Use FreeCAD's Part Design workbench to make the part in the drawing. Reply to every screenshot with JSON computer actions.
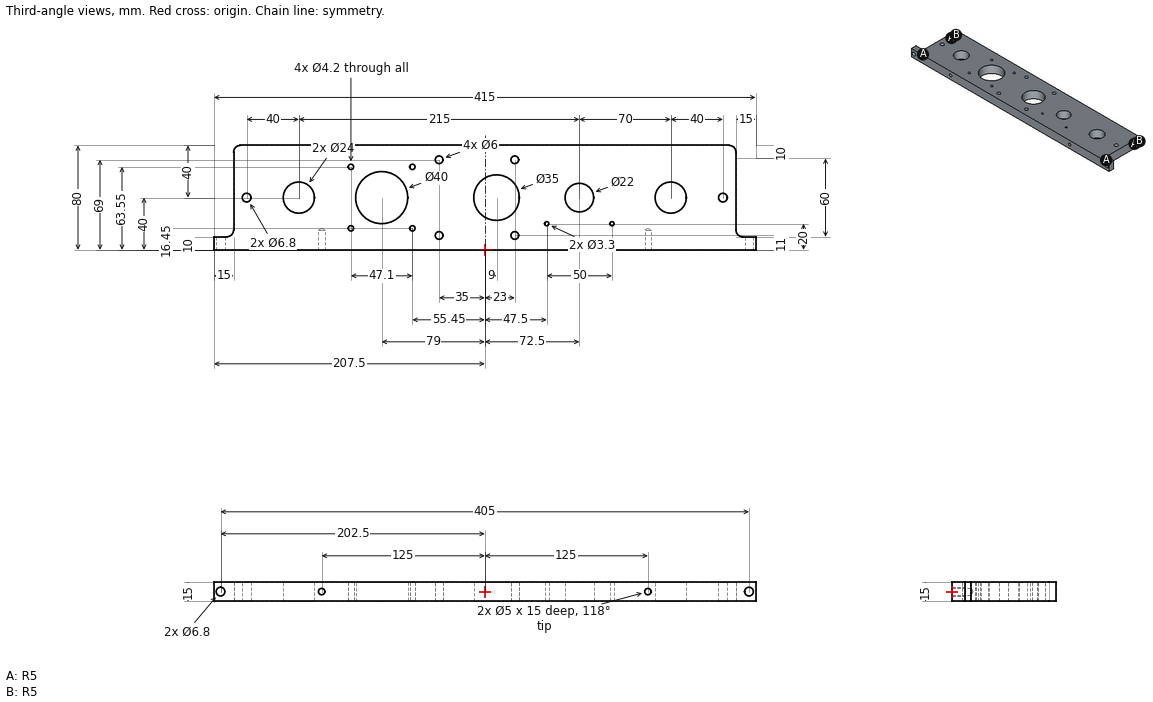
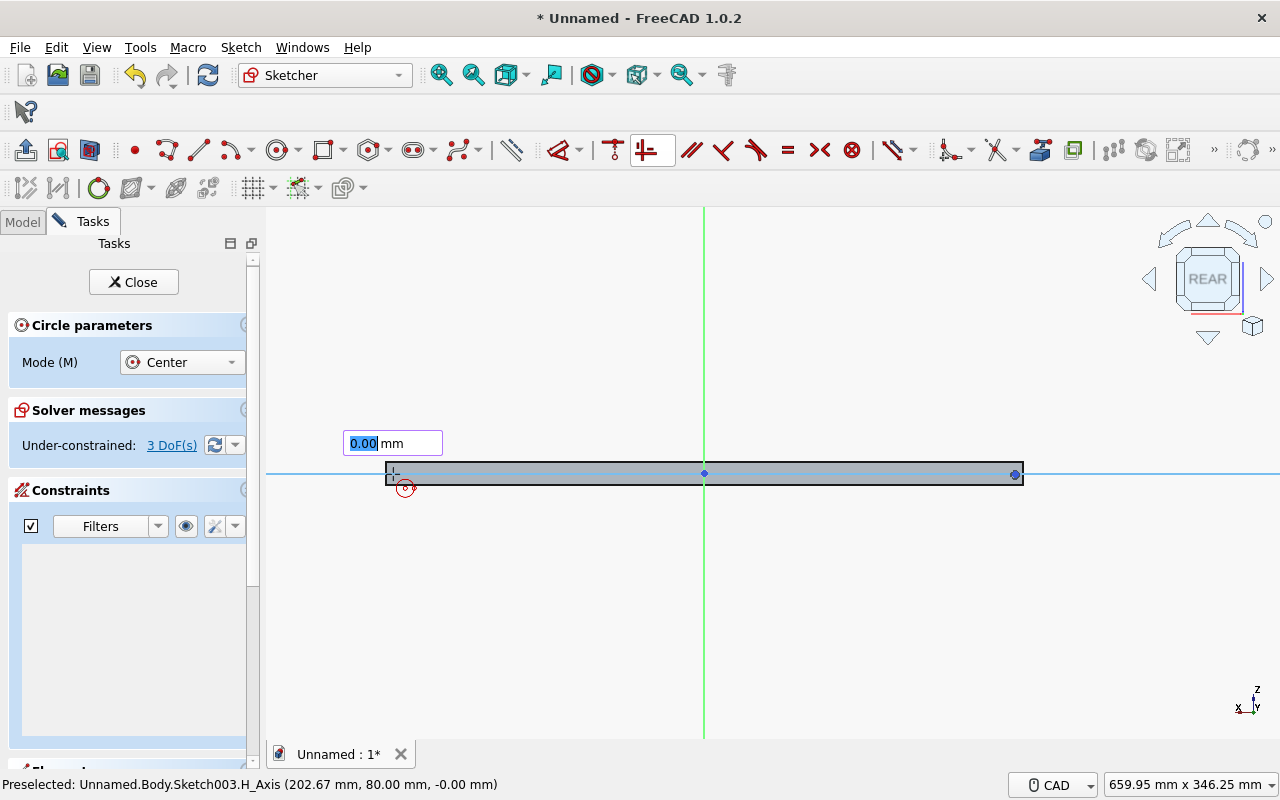
{"action": "scroll", "coordinate": [391, 479], "scroll_direction": "up", "scroll_amount": 6}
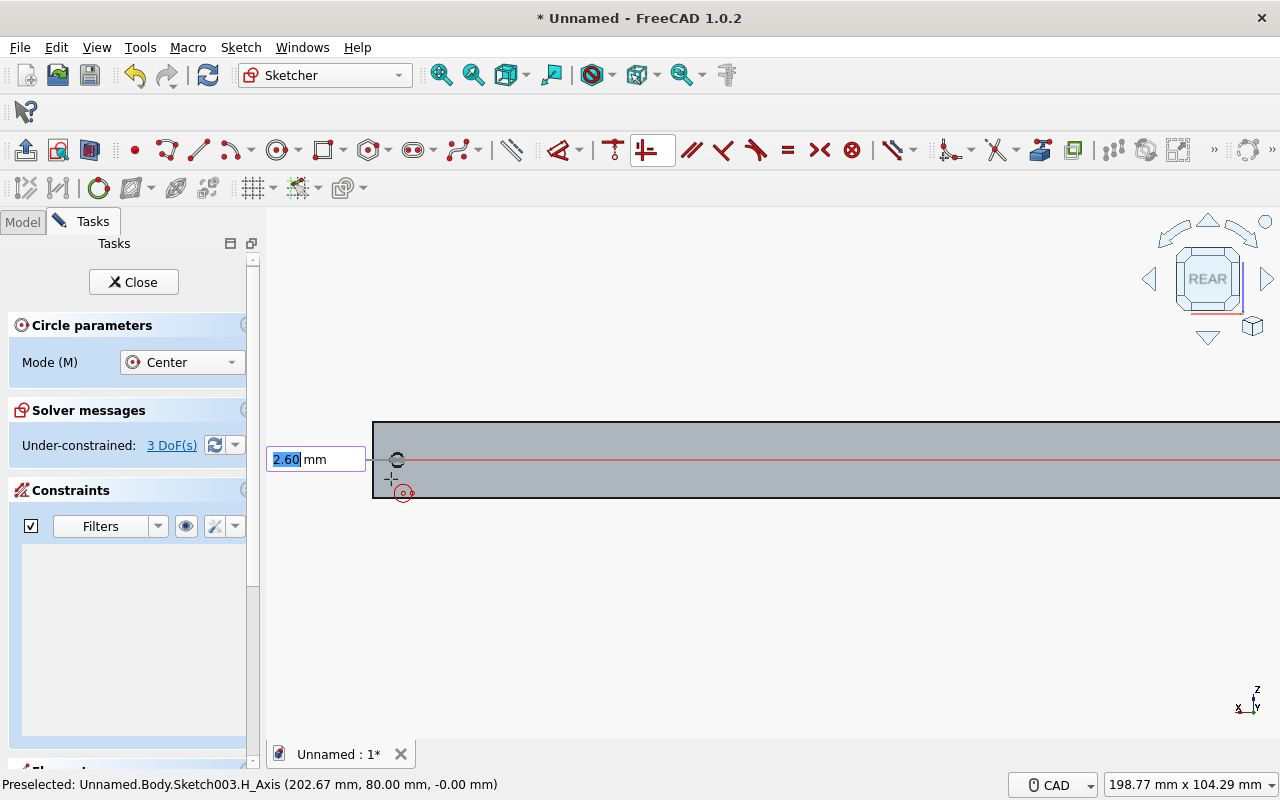
{"action": "left_click", "coordinate": [392, 476]}
{"action": "key", "text": "Escape"}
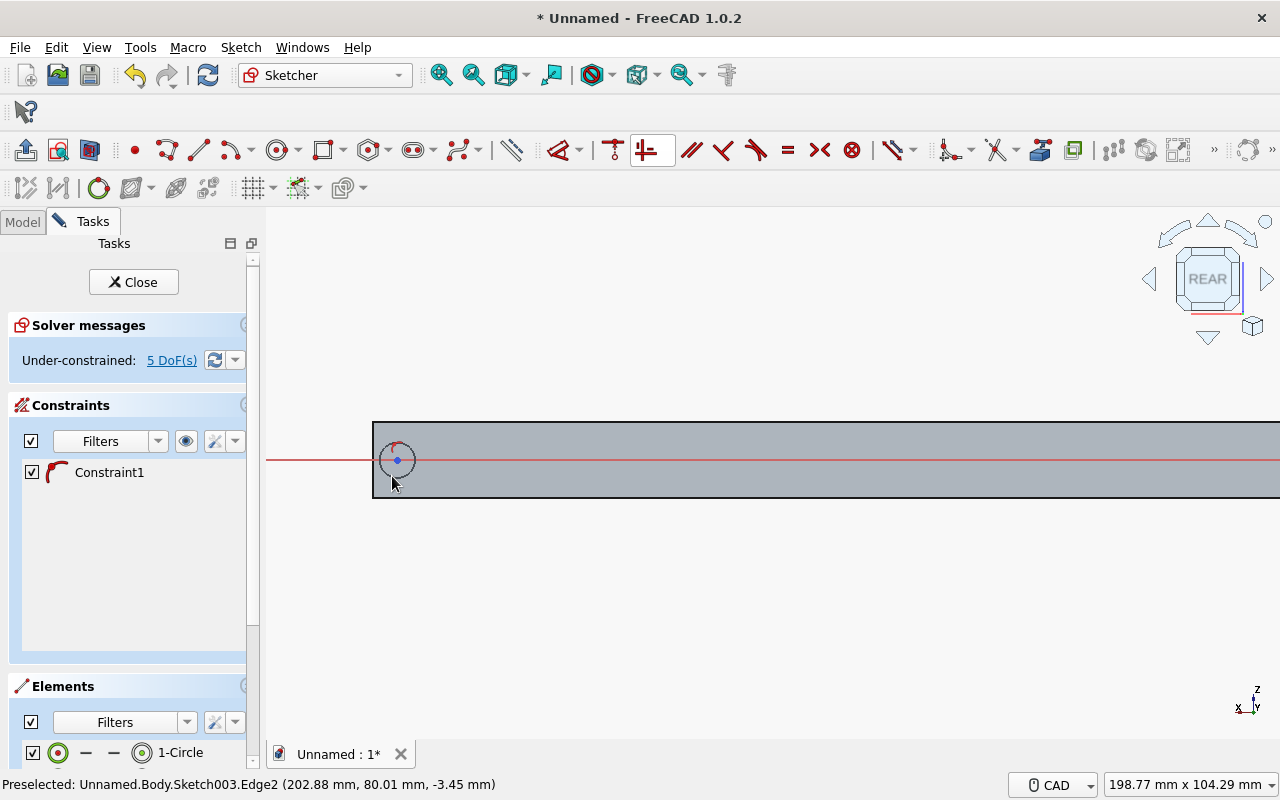
{"action": "scroll", "coordinate": [391, 479], "scroll_direction": "down", "scroll_amount": 6}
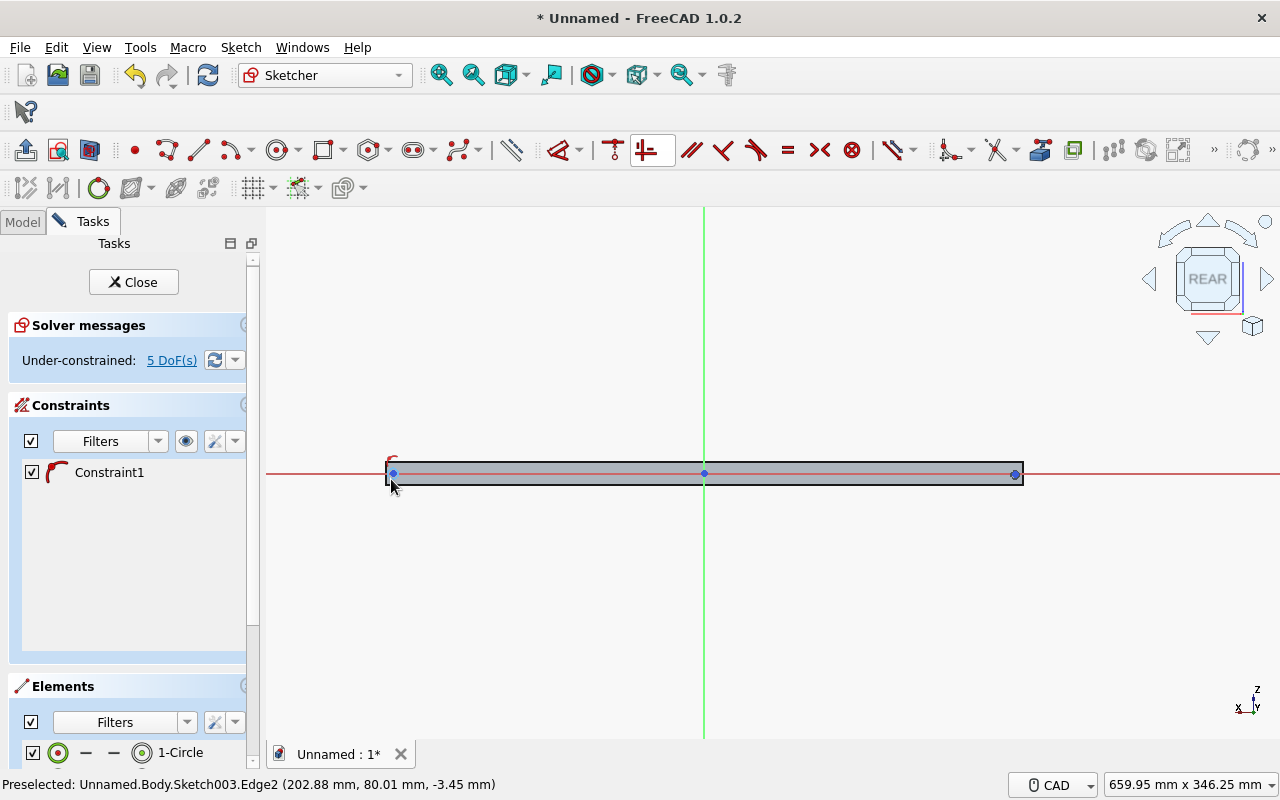
{"action": "scroll", "coordinate": [1012, 478], "scroll_direction": "up", "scroll_amount": 7}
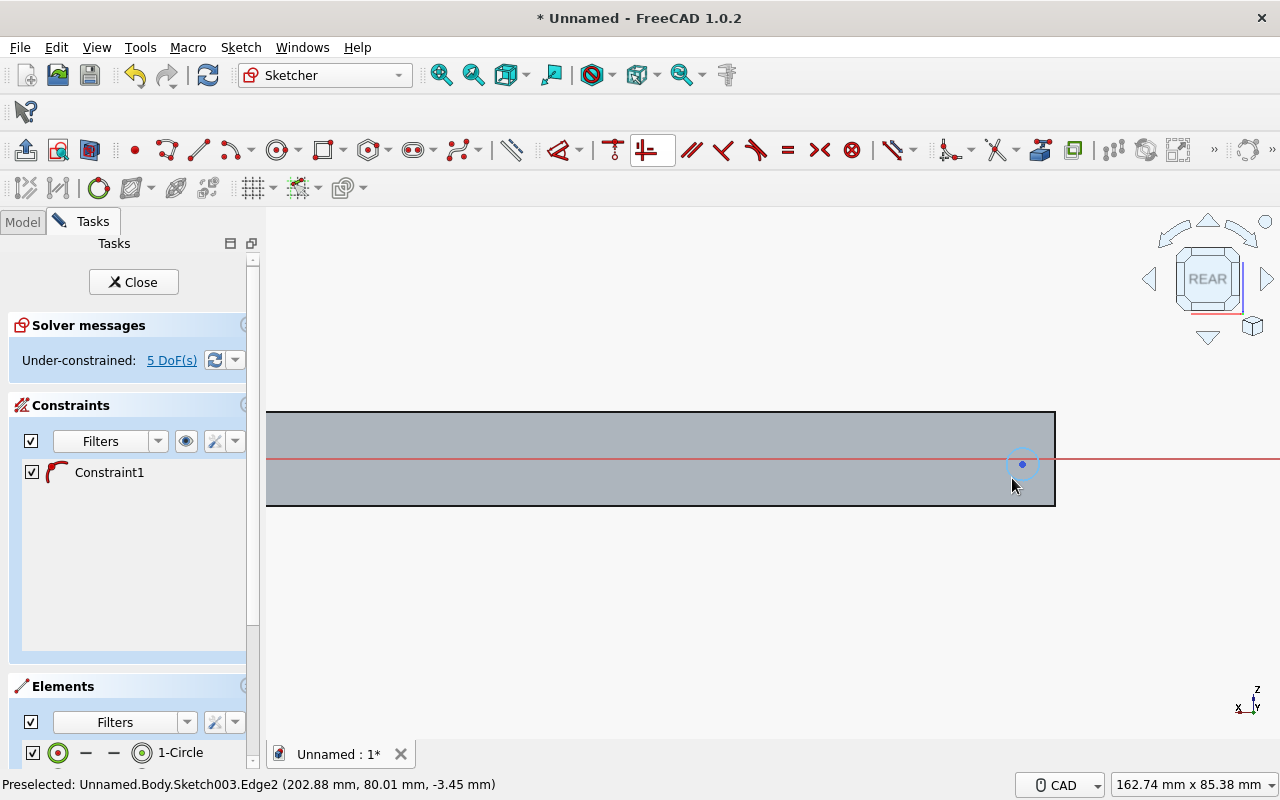
{"action": "left_click", "coordinate": [1011, 476]}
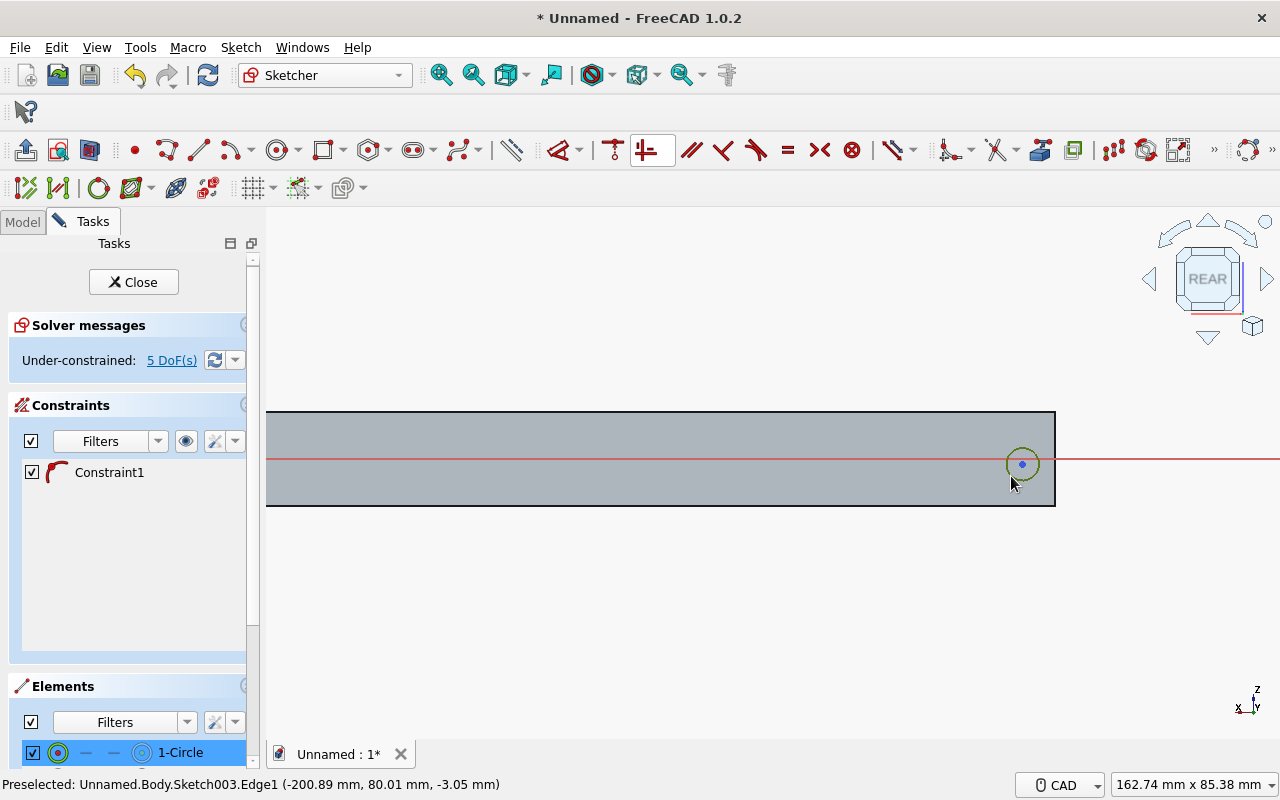
{"action": "scroll", "coordinate": [1013, 478], "scroll_direction": "down", "scroll_amount": 7}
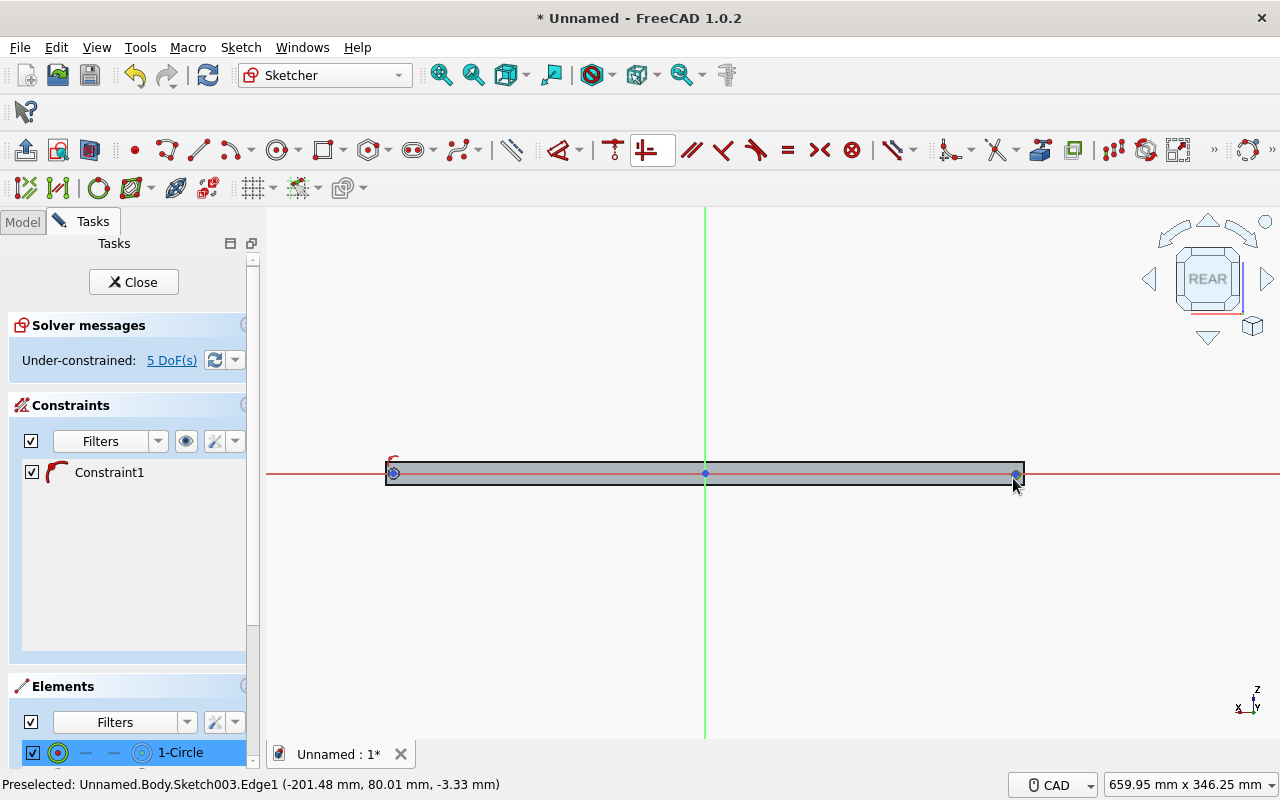
{"action": "scroll", "coordinate": [398, 470], "scroll_direction": "up", "scroll_amount": 7}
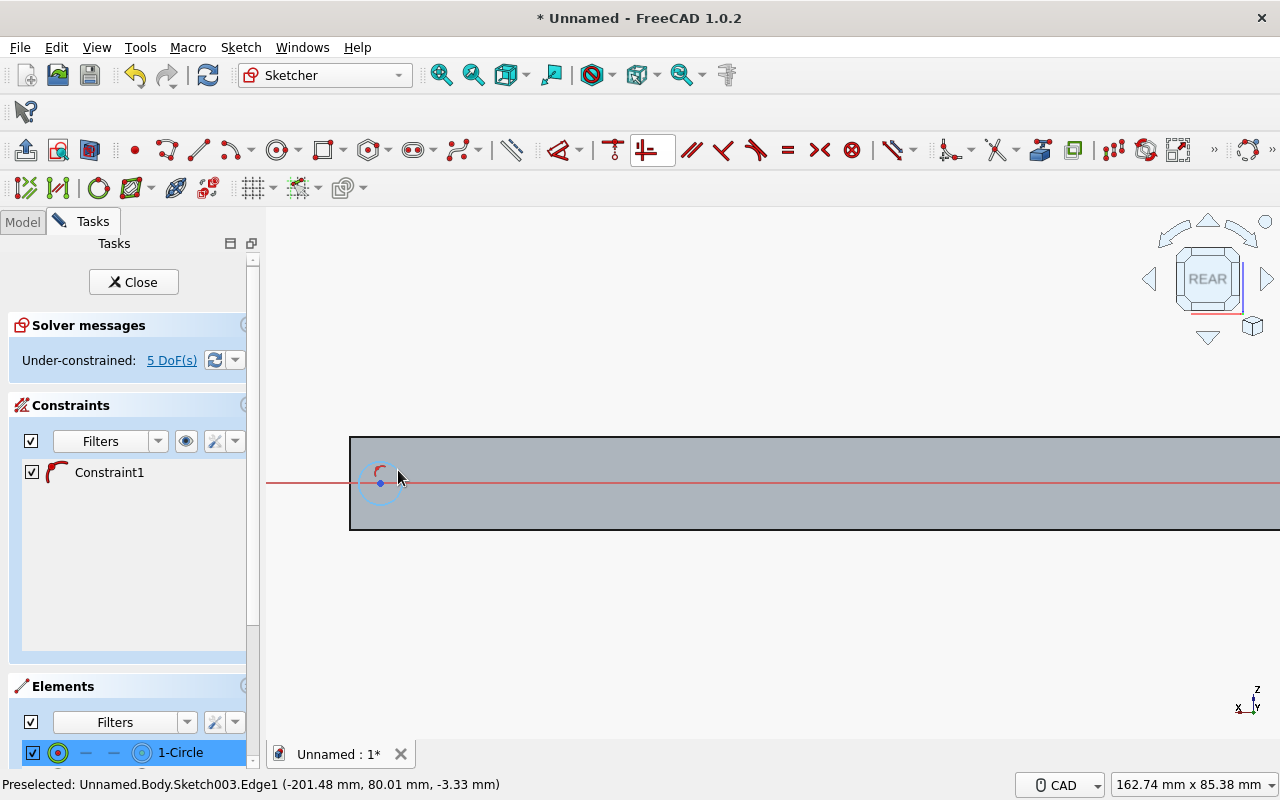
{"action": "left_click", "coordinate": [396, 468]}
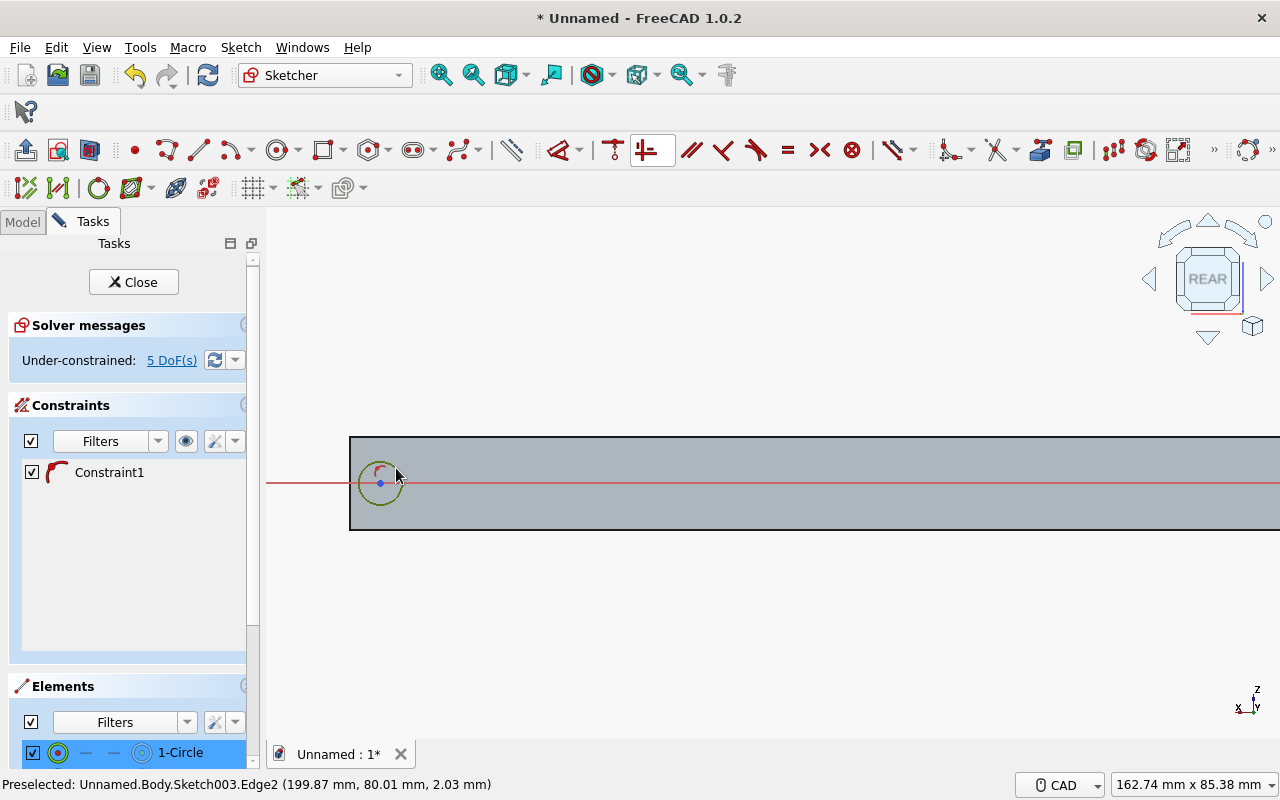
{"action": "left_click", "coordinate": [788, 150]}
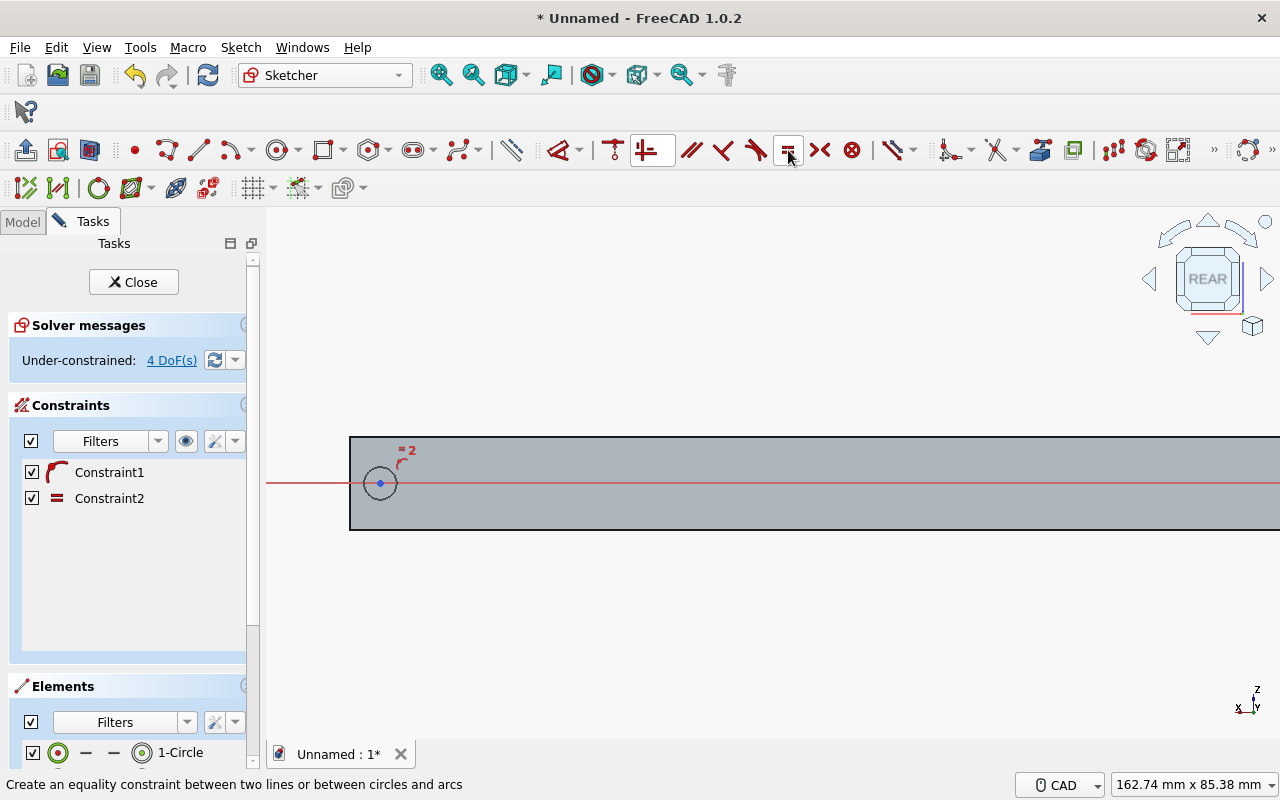
{"action": "scroll", "coordinate": [397, 470], "scroll_direction": "down", "scroll_amount": 7}